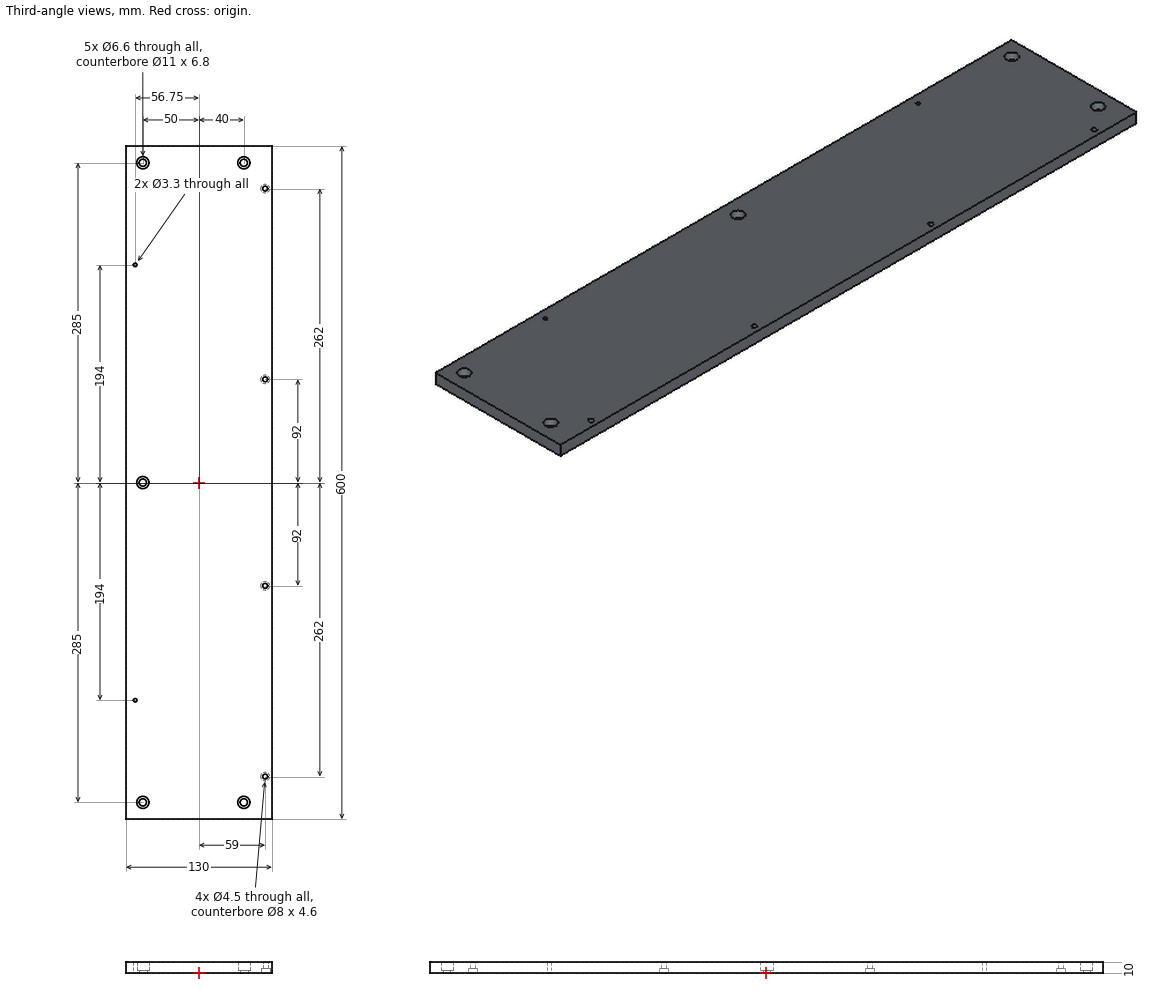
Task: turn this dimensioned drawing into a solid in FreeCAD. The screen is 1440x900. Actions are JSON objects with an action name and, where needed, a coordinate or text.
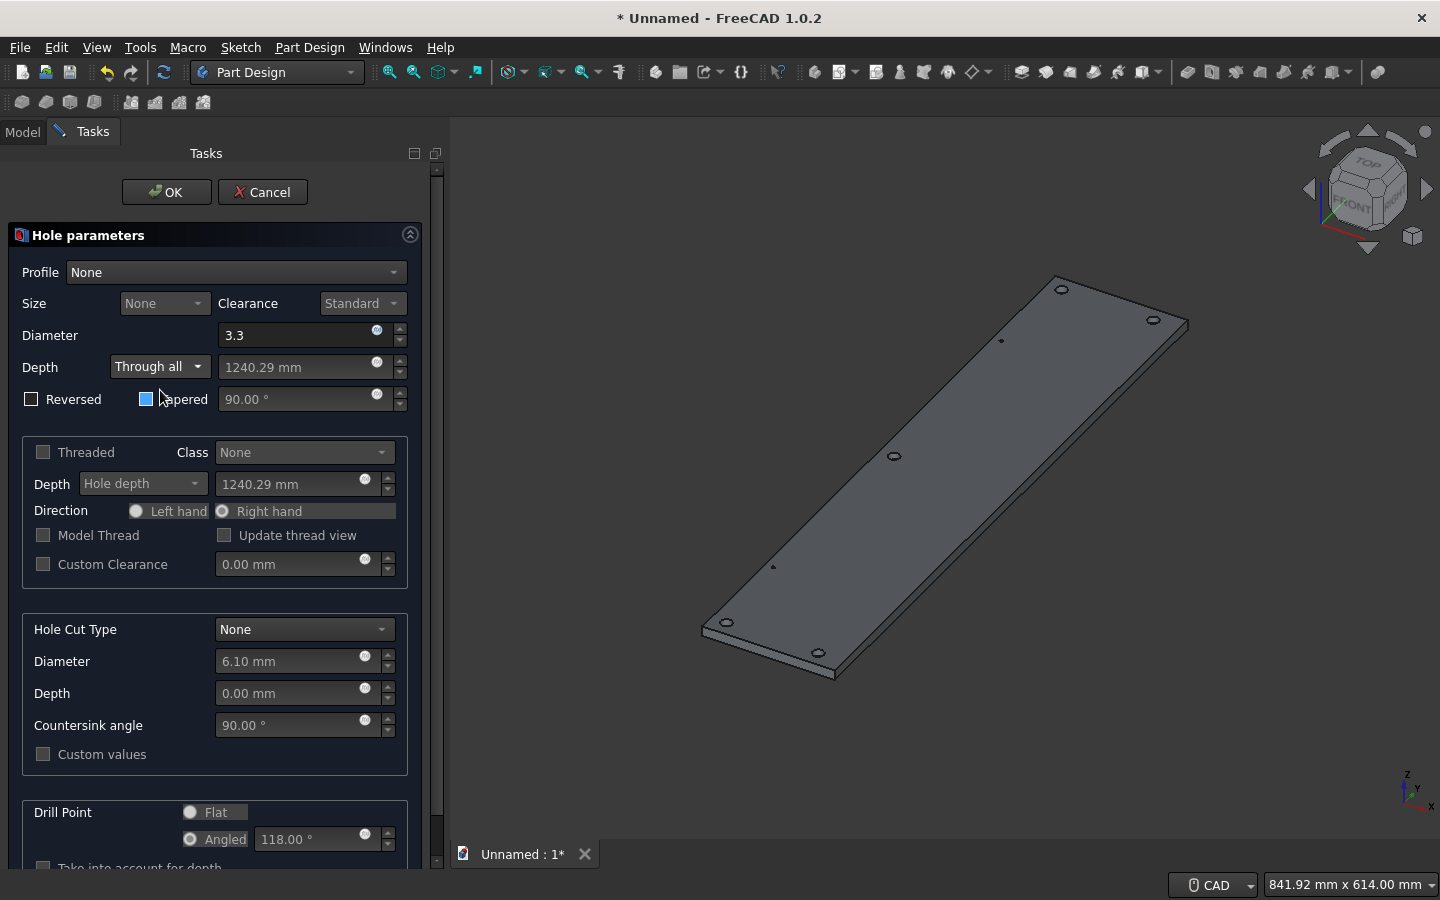
{"action": "left_click", "coordinate": [167, 192]}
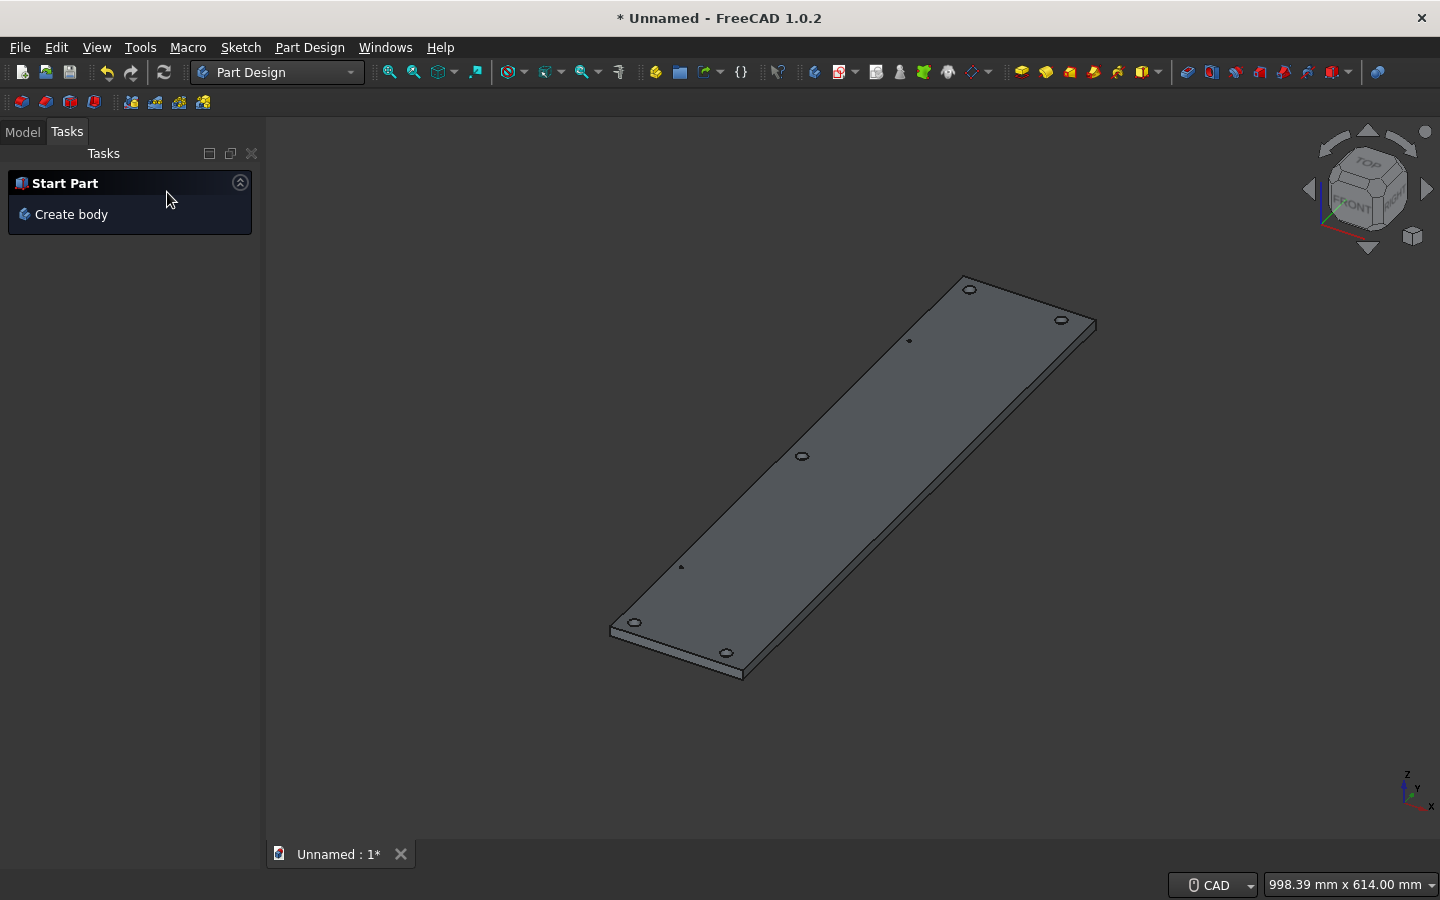
{"action": "key", "text": "5"}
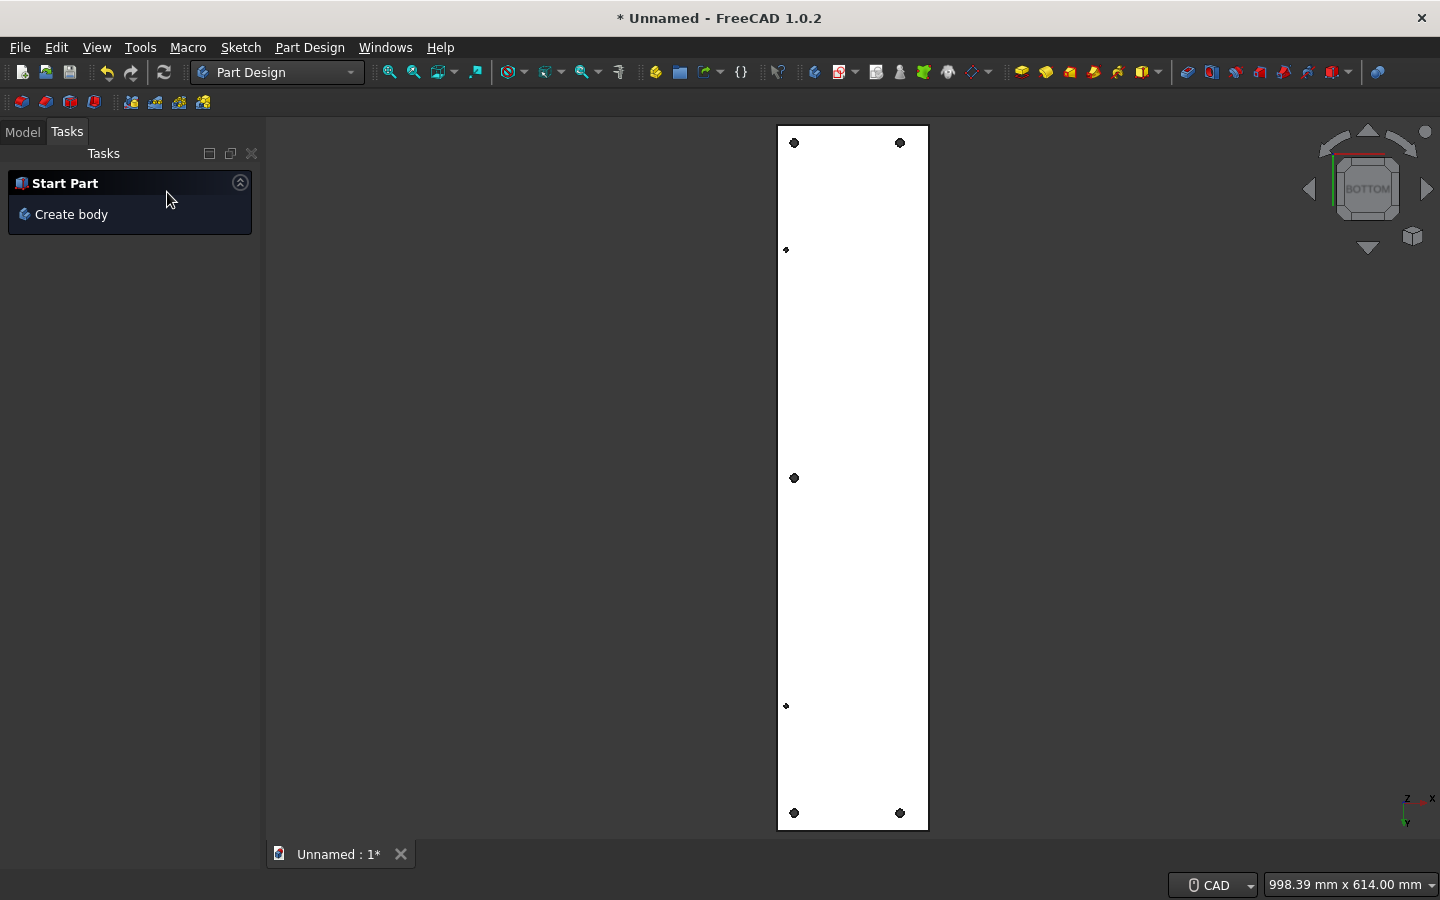
{"action": "left_click", "coordinate": [853, 578]}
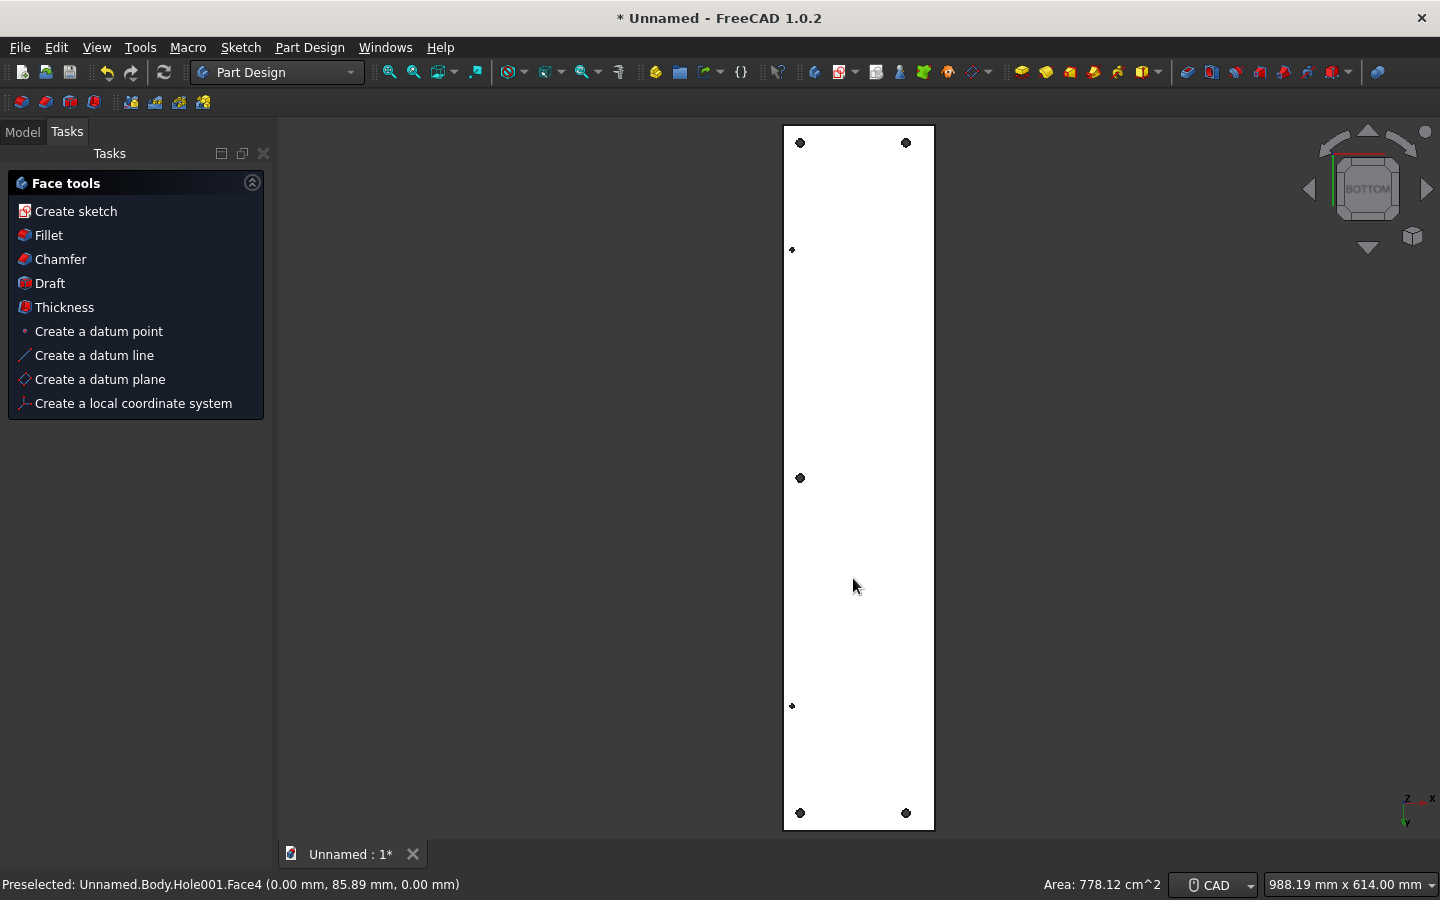
{"action": "left_click", "coordinate": [840, 72]}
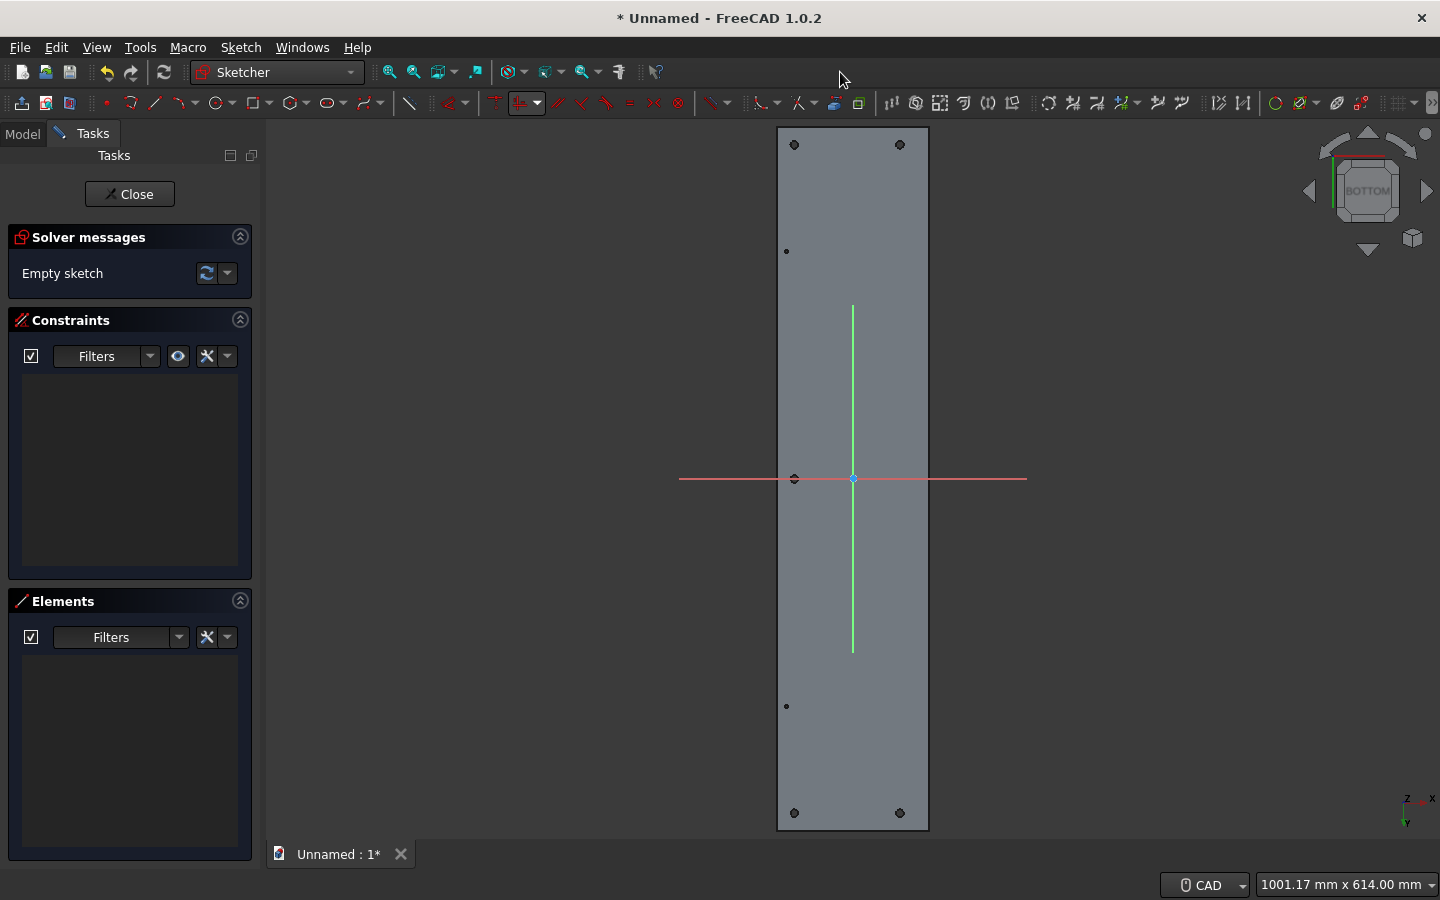
{"action": "scroll", "coordinate": [313, 479], "scroll_direction": "down", "scroll_amount": 1}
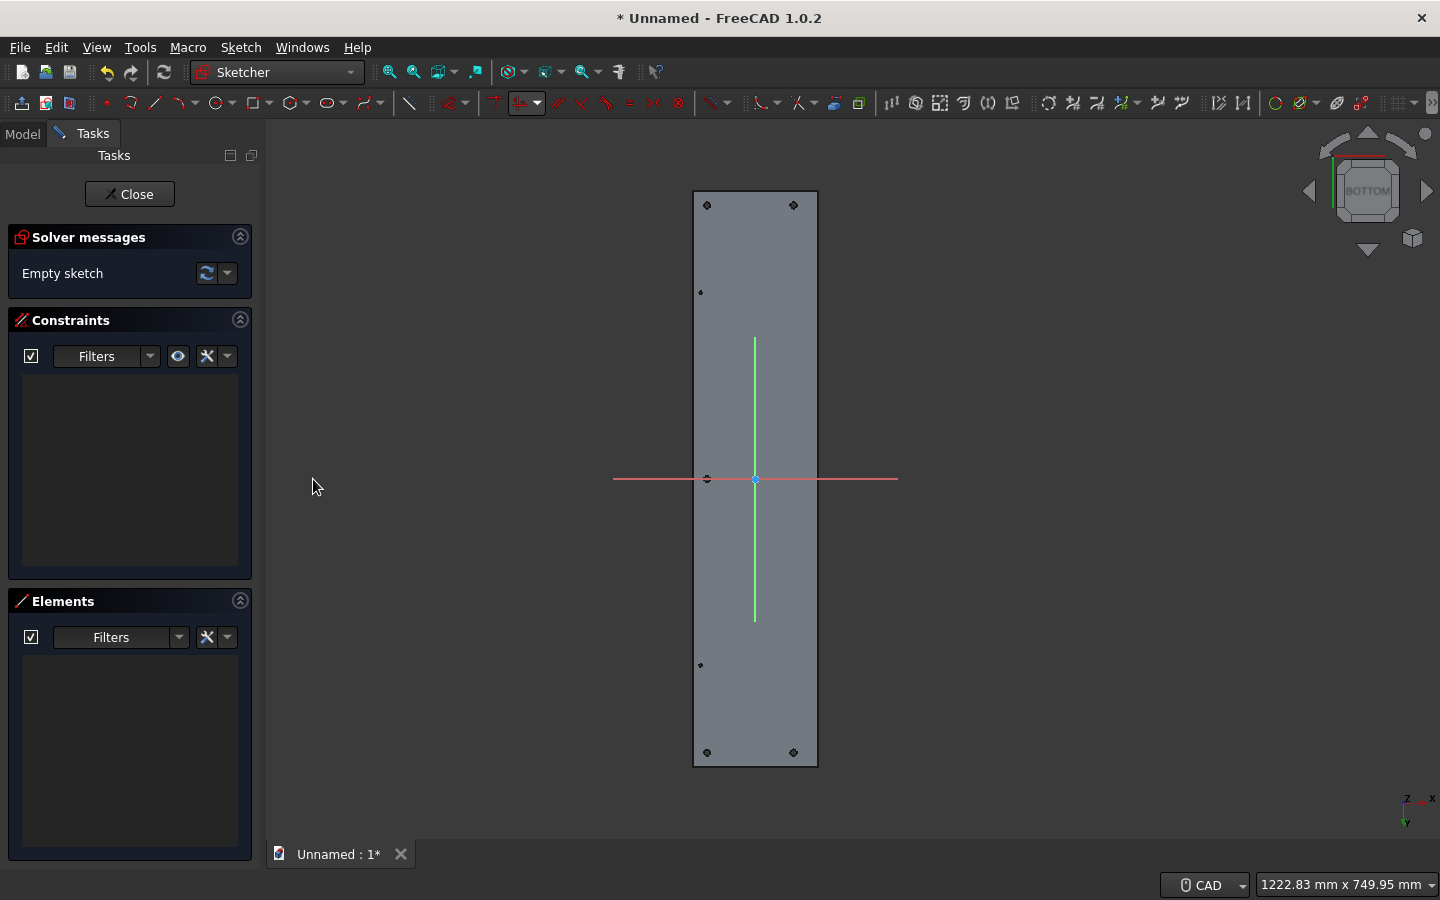
{"action": "left_click", "coordinate": [216, 104]}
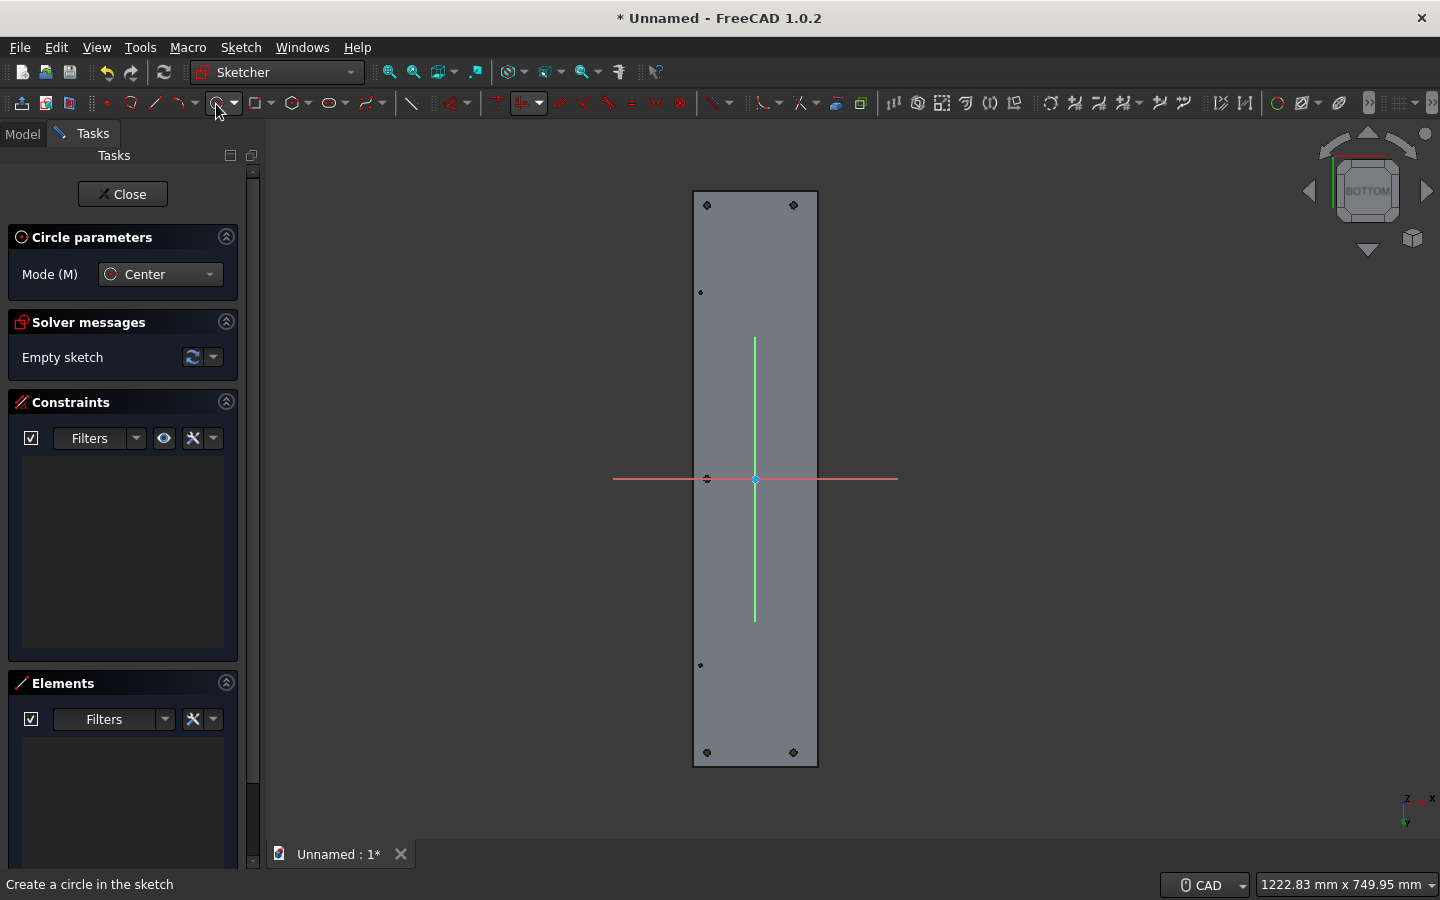
{"action": "scroll", "coordinate": [812, 228], "scroll_direction": "up", "scroll_amount": 12}